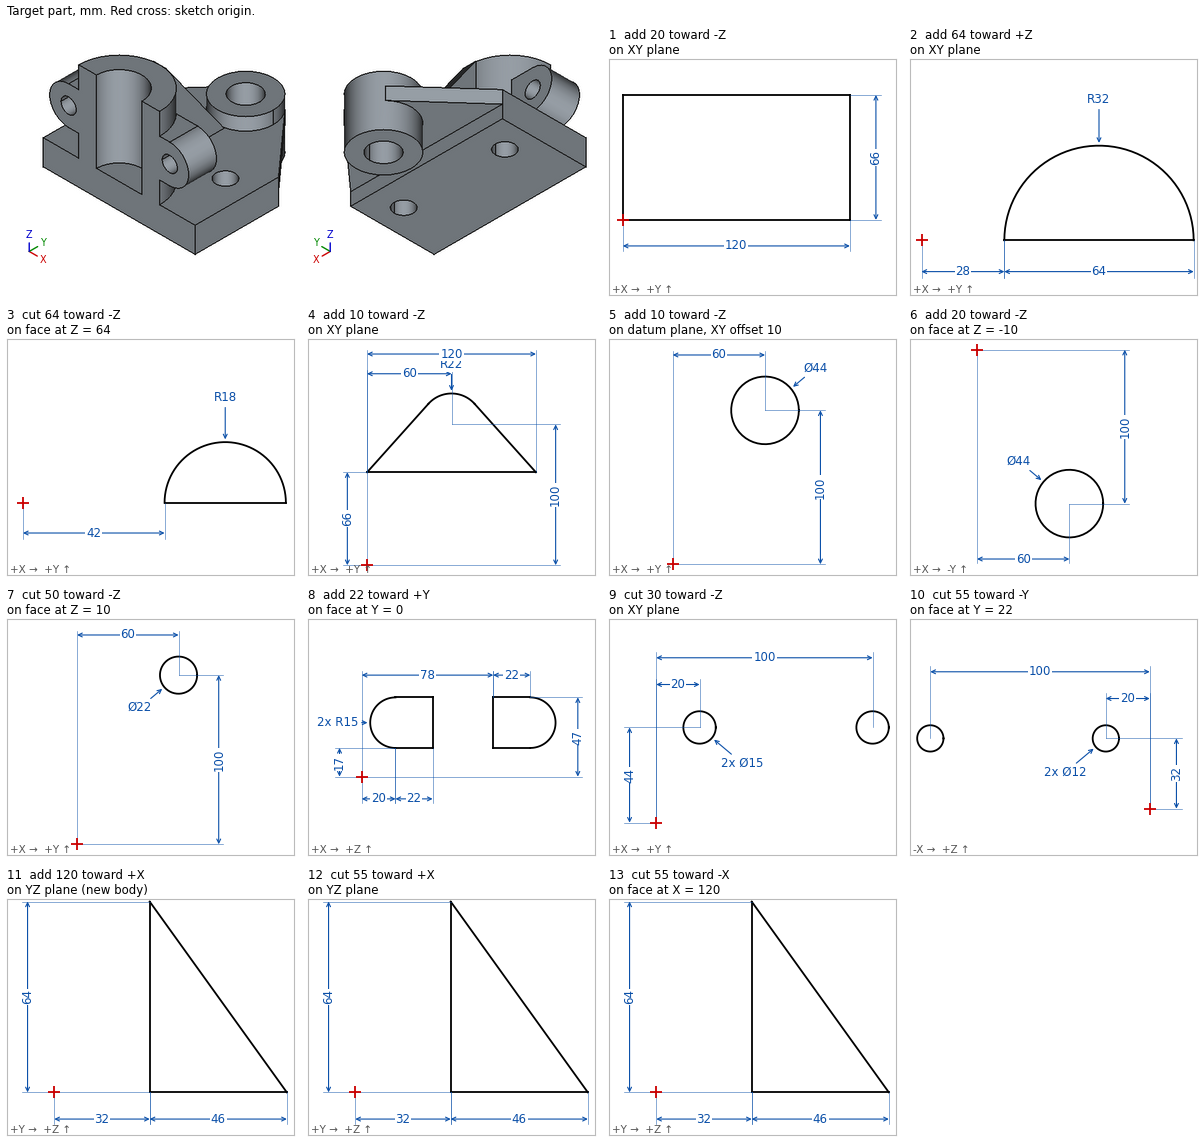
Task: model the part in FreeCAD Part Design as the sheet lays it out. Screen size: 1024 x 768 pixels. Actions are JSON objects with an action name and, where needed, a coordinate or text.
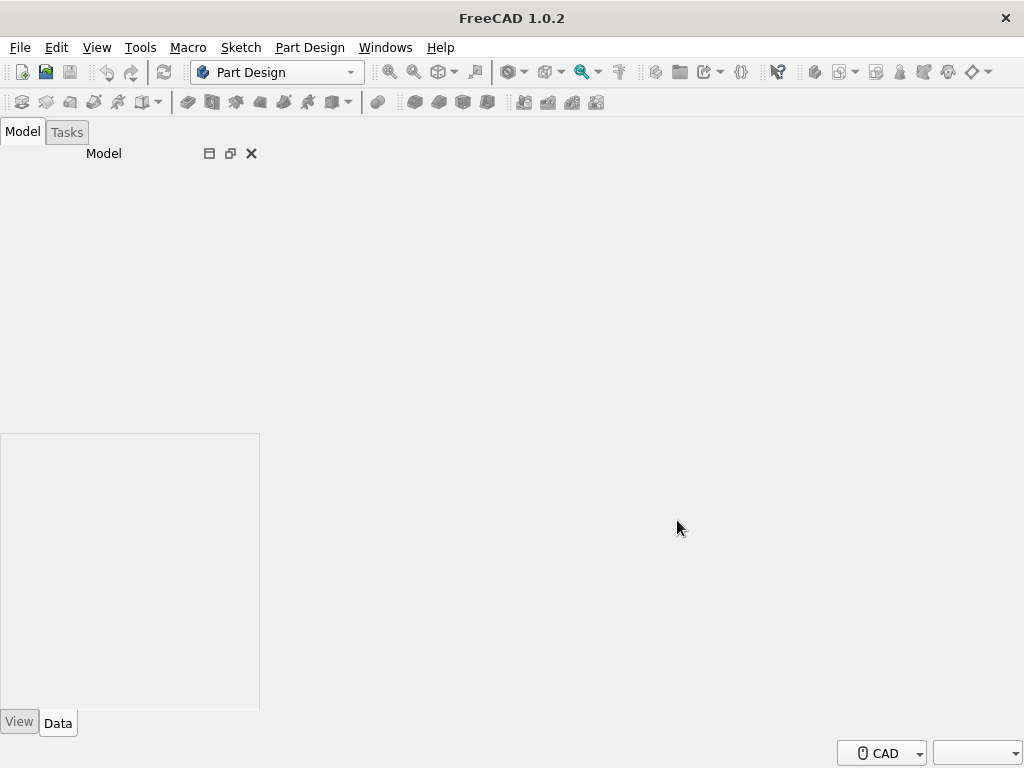
{"action": "left_click", "coordinate": [22, 72]}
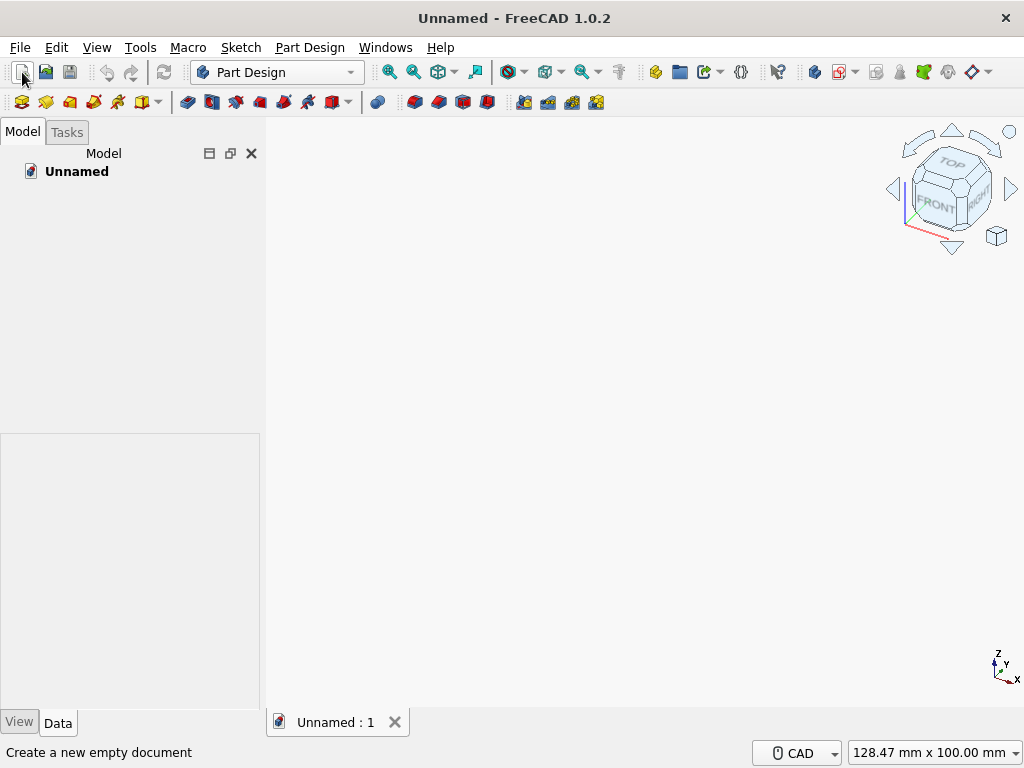
{"action": "left_click", "coordinate": [840, 72]}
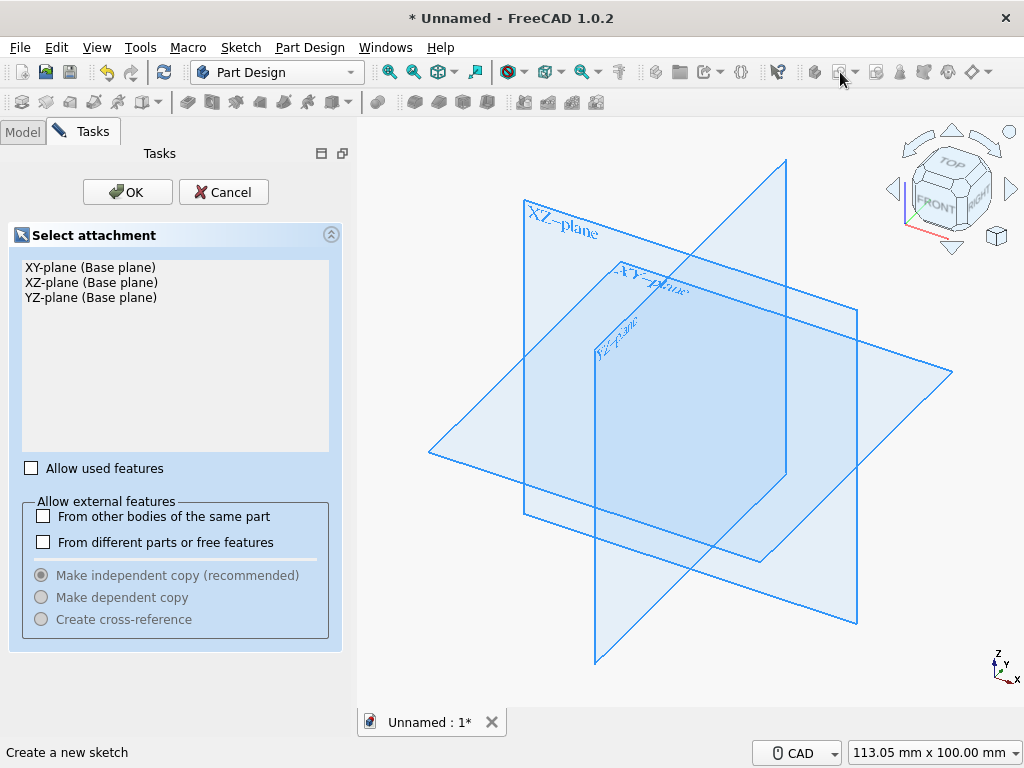
{"action": "left_click", "coordinate": [82, 268]}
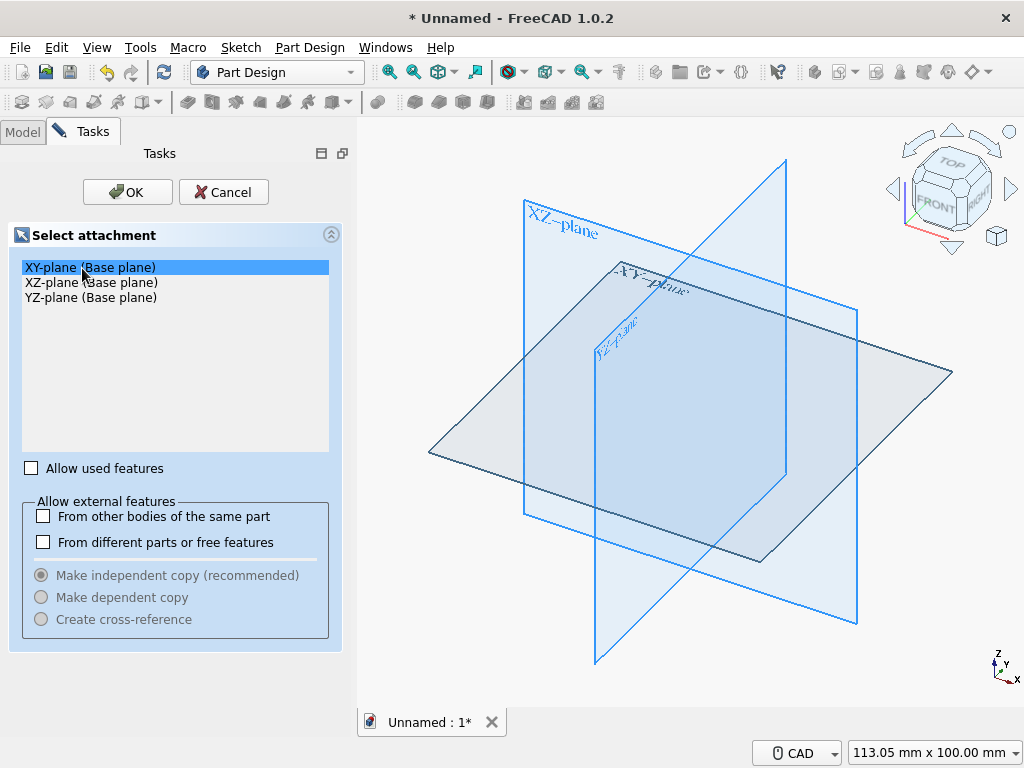
{"action": "left_click", "coordinate": [128, 192]}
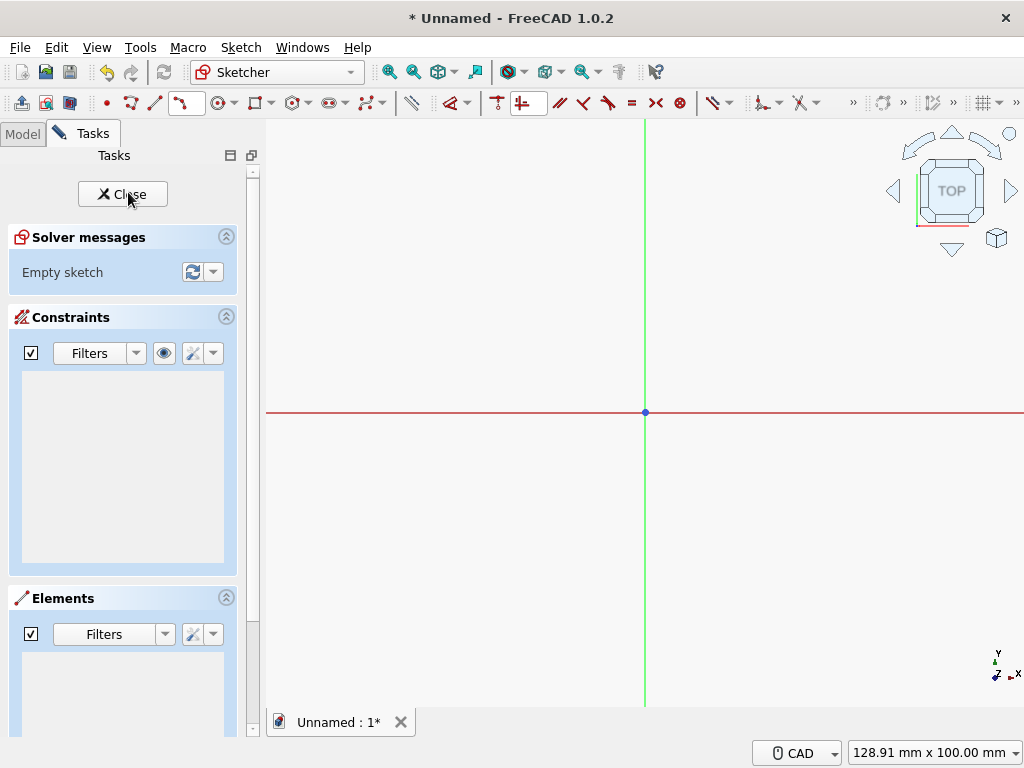
{"action": "scroll", "coordinate": [294, 571], "scroll_direction": "down", "scroll_amount": 4}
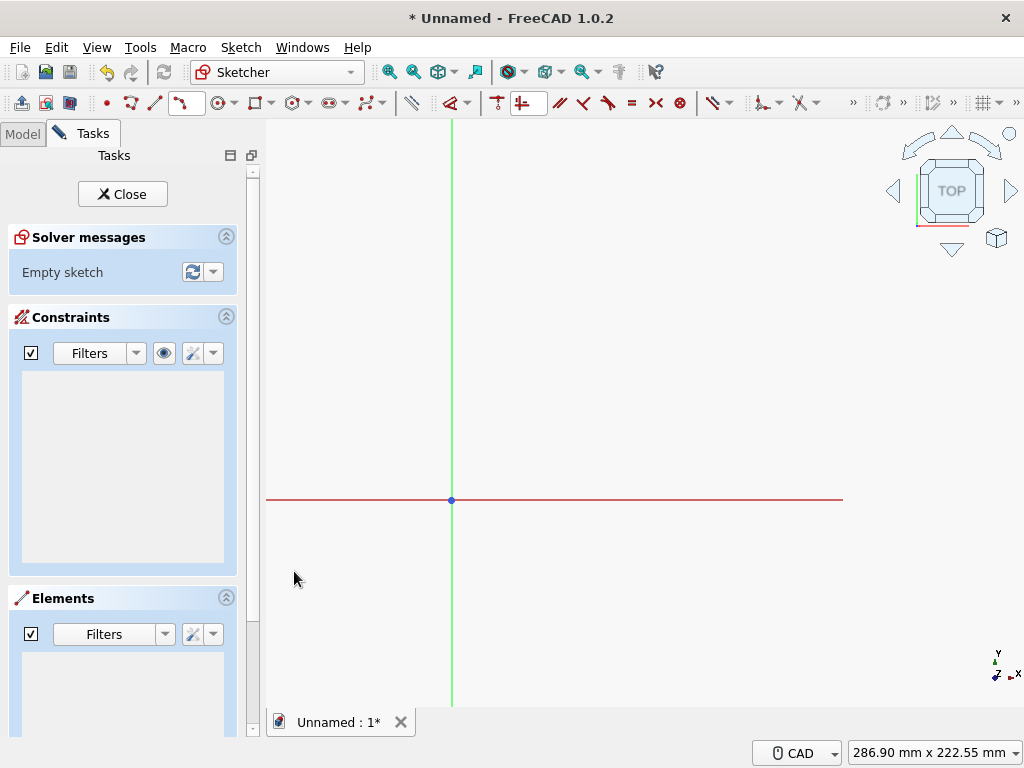
{"action": "left_click", "coordinate": [256, 104]}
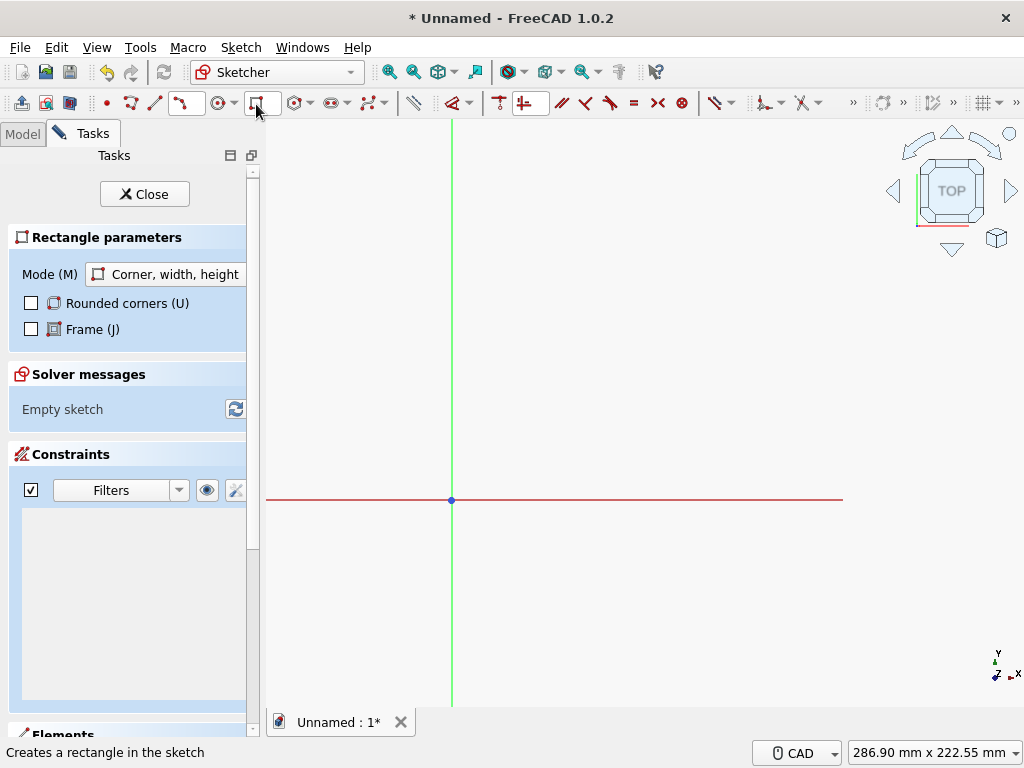
{"action": "left_click", "coordinate": [452, 500]}
{"action": "left_click", "coordinate": [769, 326]}
{"action": "key", "text": "Escape"}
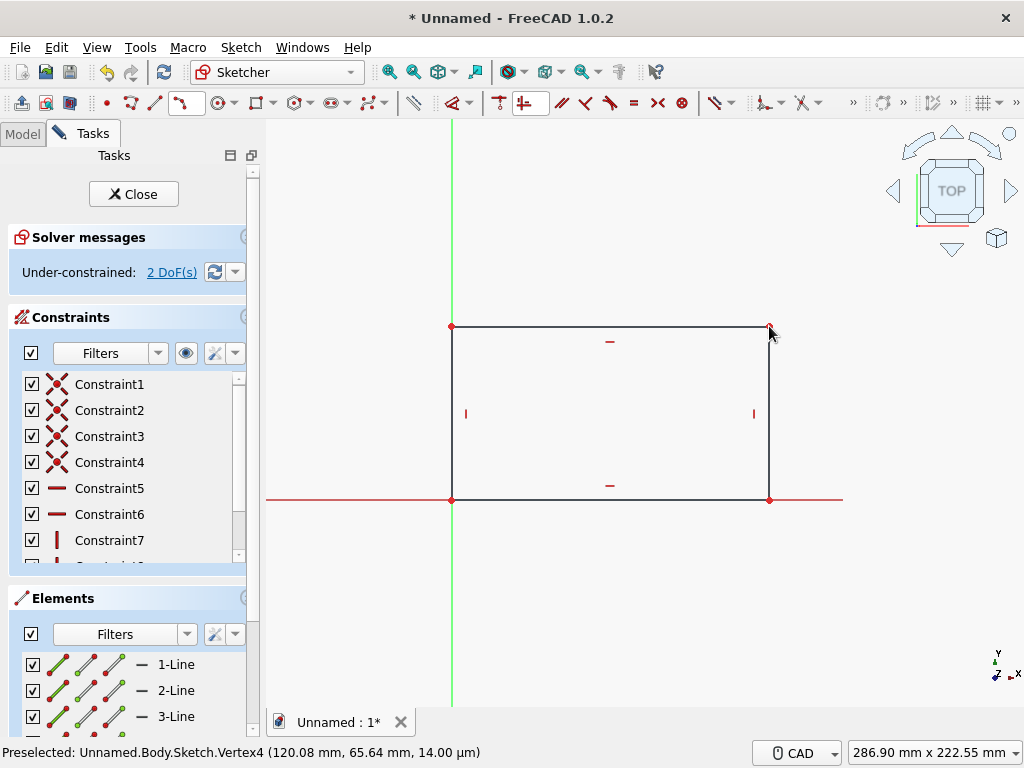
{"action": "left_click", "coordinate": [452, 104]}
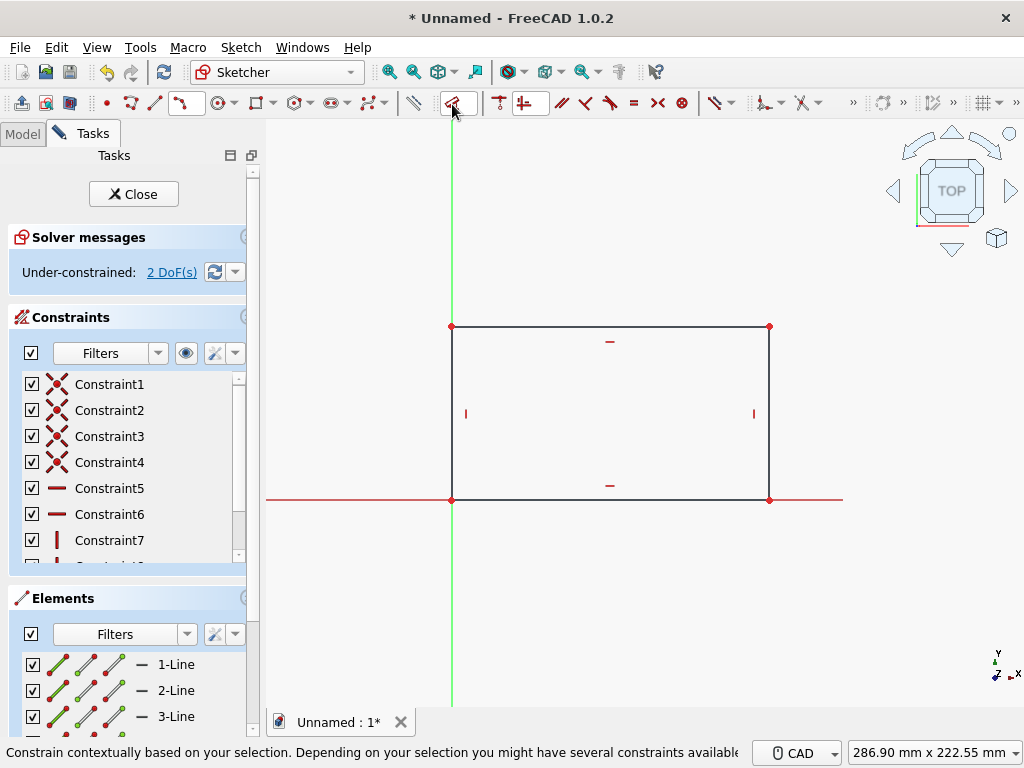
{"action": "left_click", "coordinate": [769, 448]}
{"action": "left_click", "coordinate": [803, 414]}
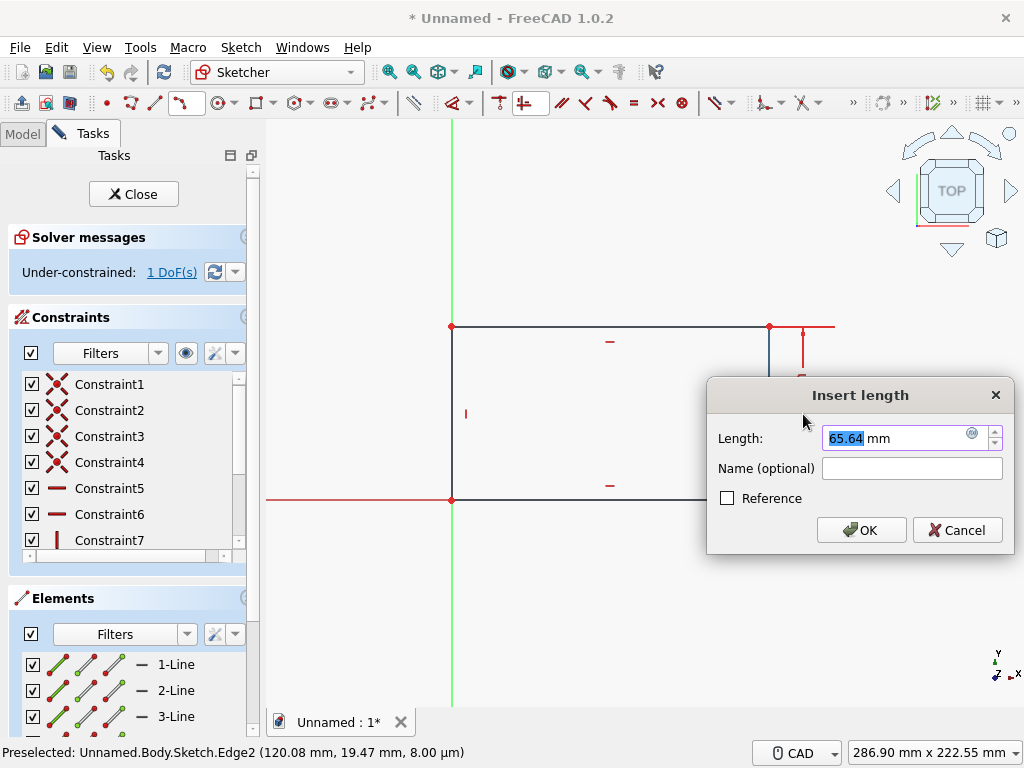
{"action": "type", "text": "66"}
{"action": "key", "text": "Return"}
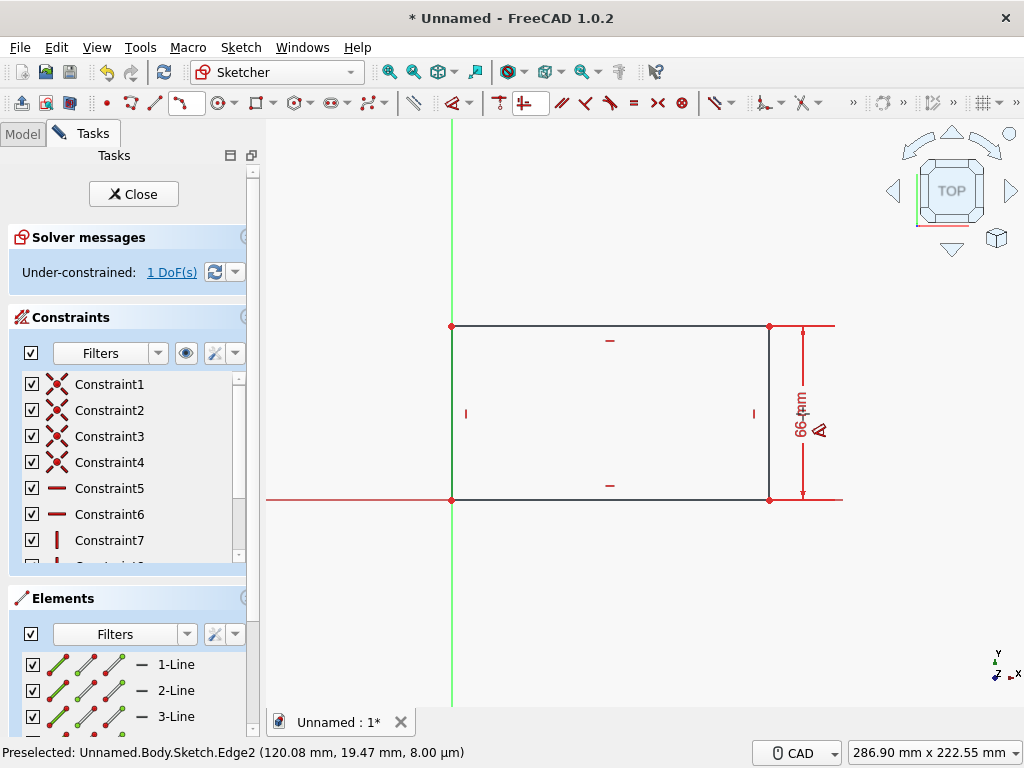
{"action": "left_click", "coordinate": [547, 500]}
{"action": "left_click", "coordinate": [610, 534]}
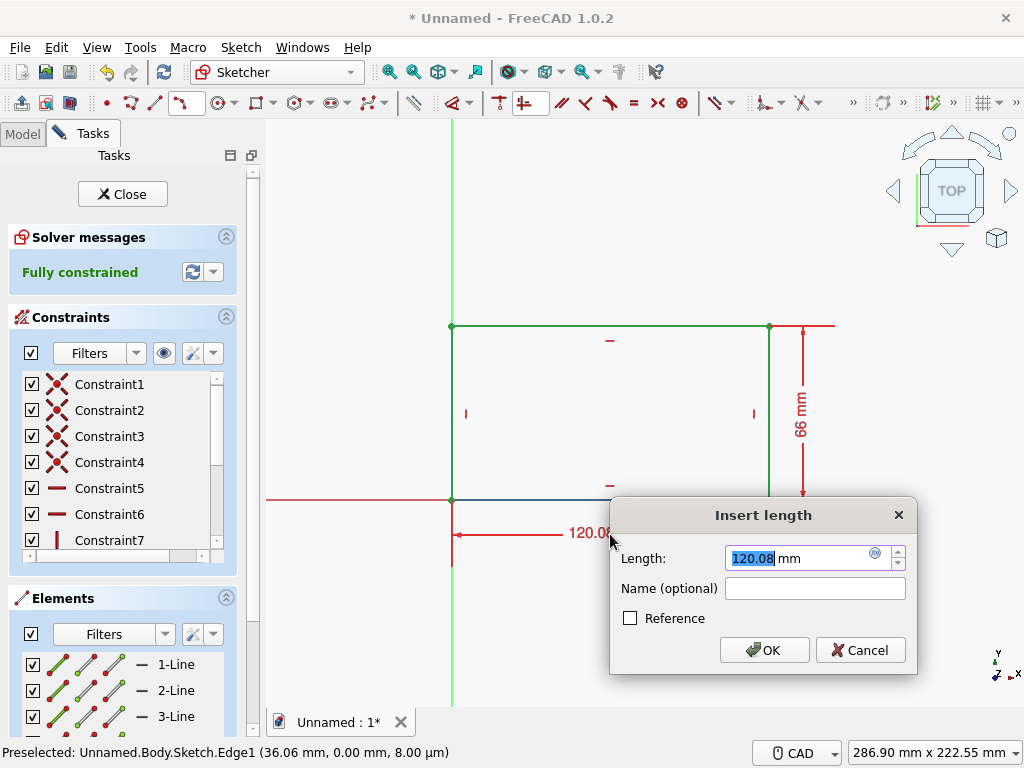
{"action": "type", "text": "120"}
{"action": "key", "text": "Return"}
{"action": "key", "text": "Escape"}